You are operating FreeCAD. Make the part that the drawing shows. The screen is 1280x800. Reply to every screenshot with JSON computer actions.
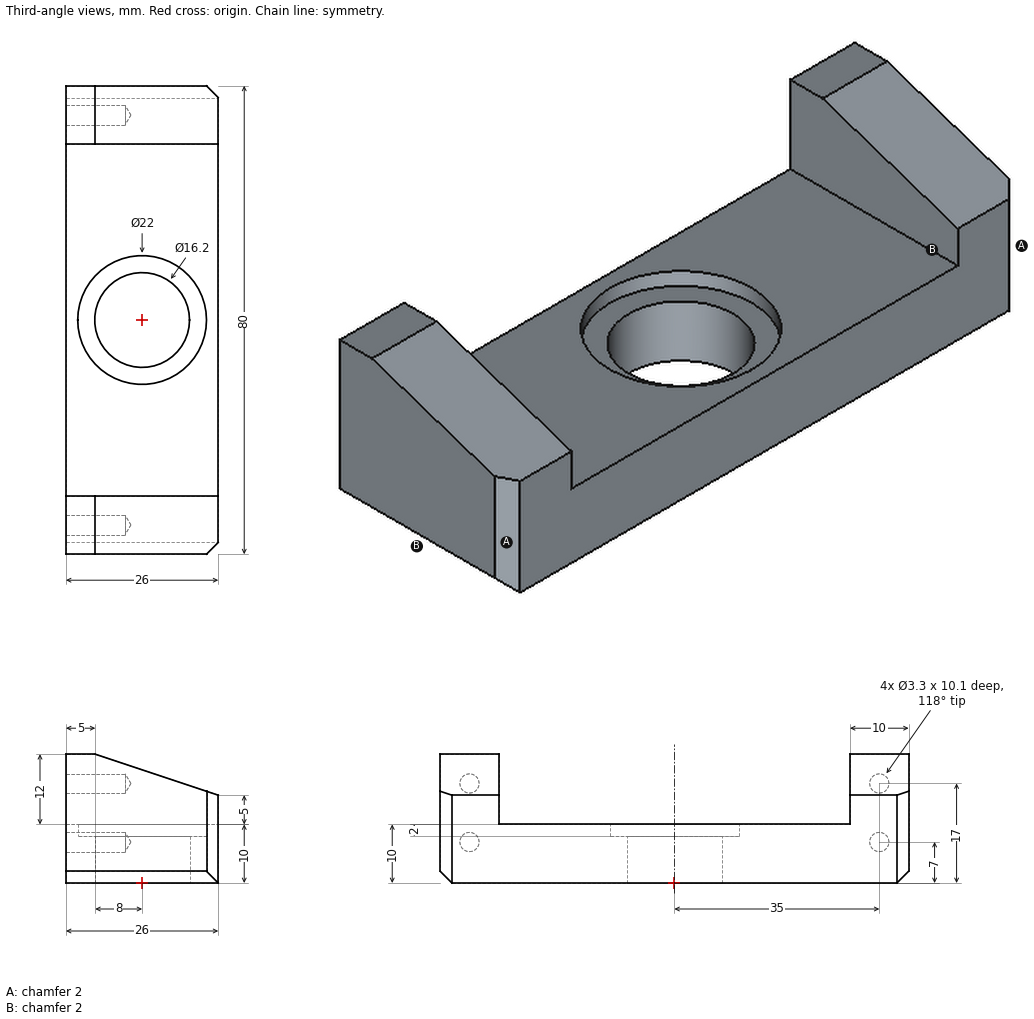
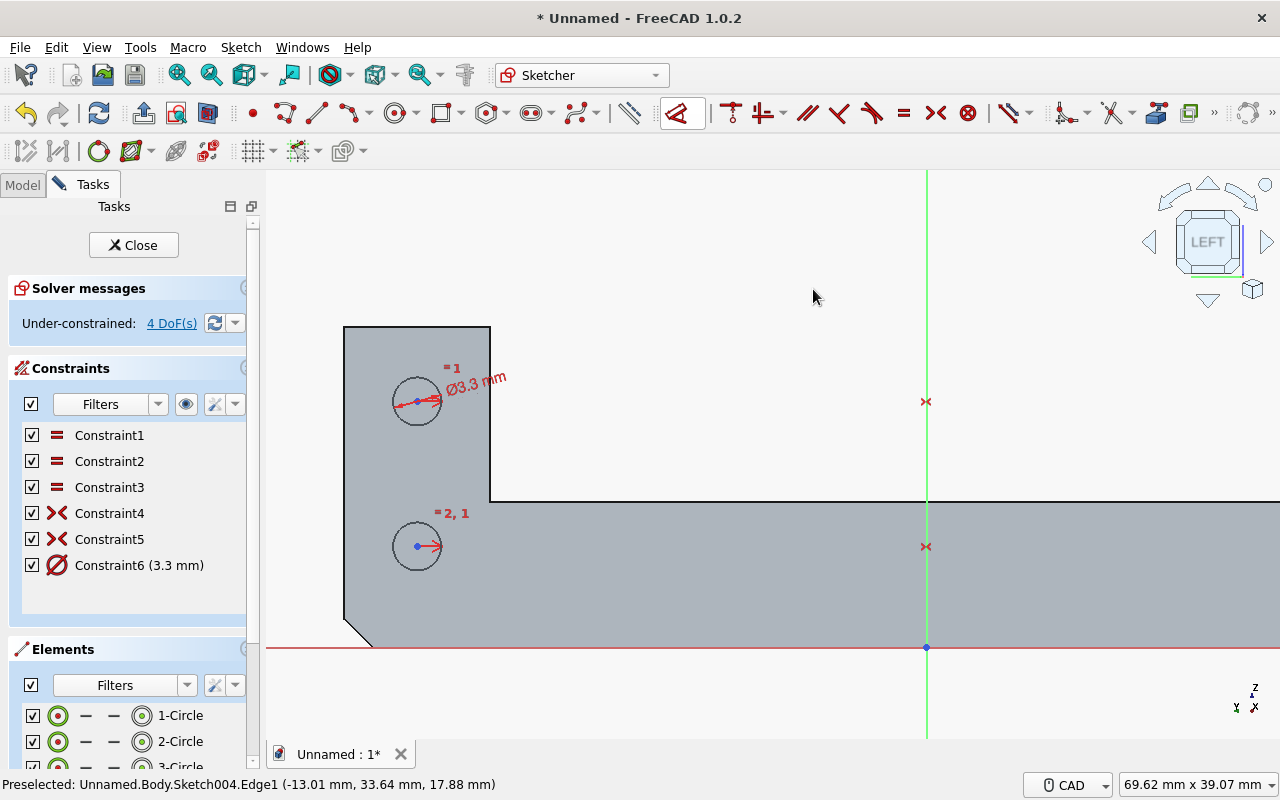
{"action": "left_click", "coordinate": [417, 546]}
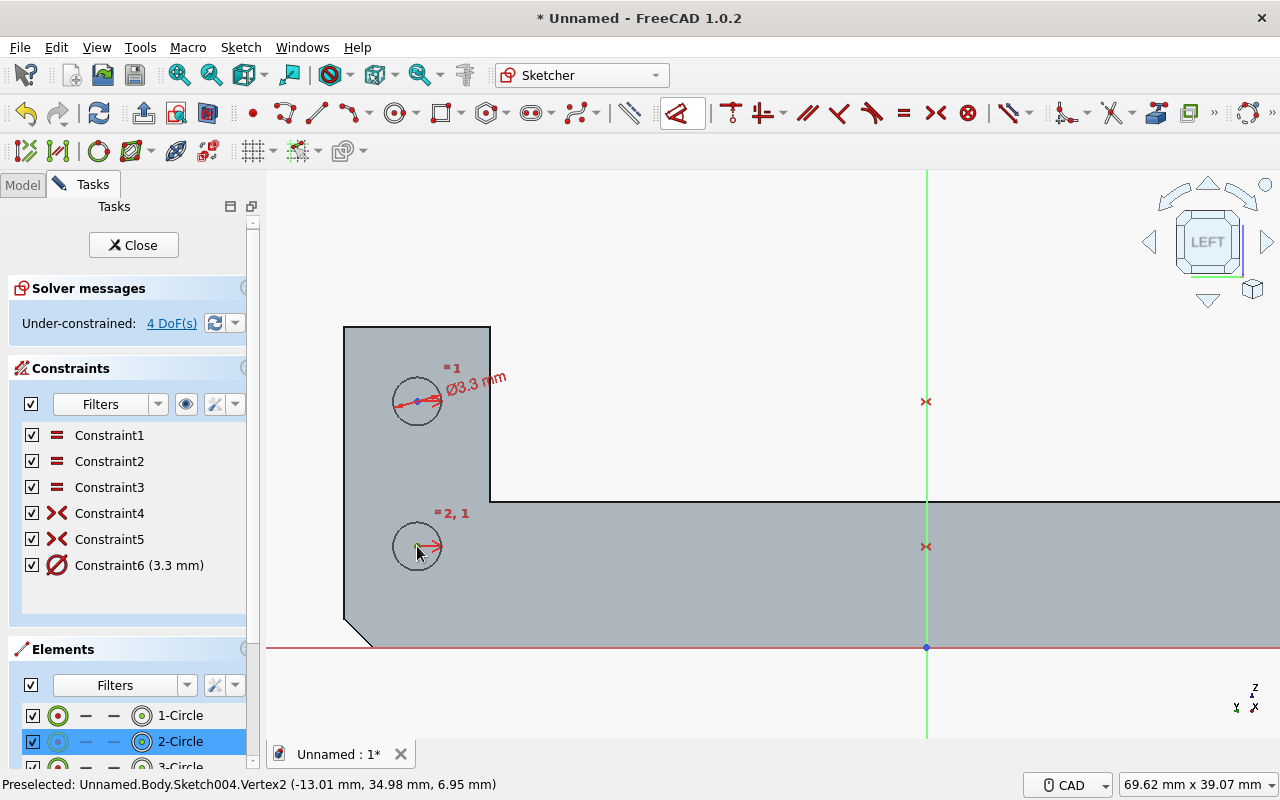
{"action": "key", "text": "i"}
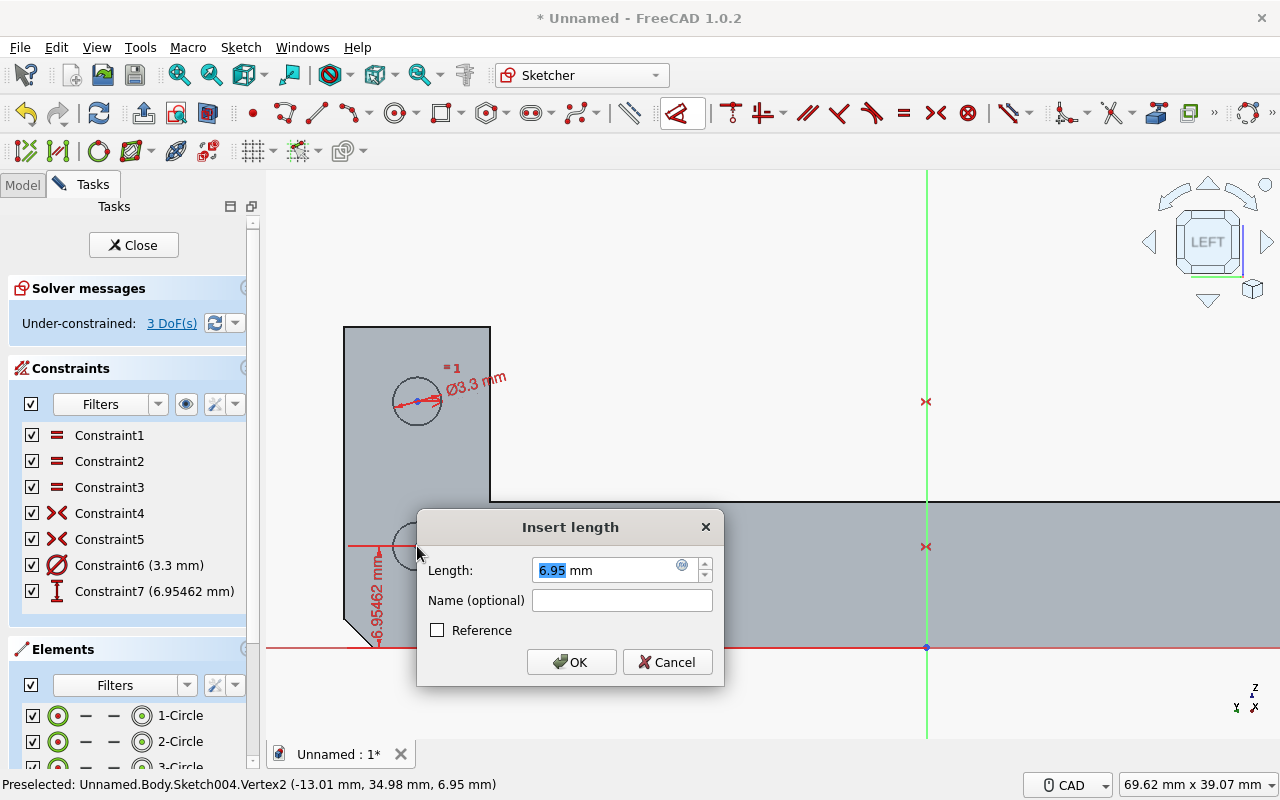
{"action": "type", "text": "7"}
{"action": "key", "text": "Return"}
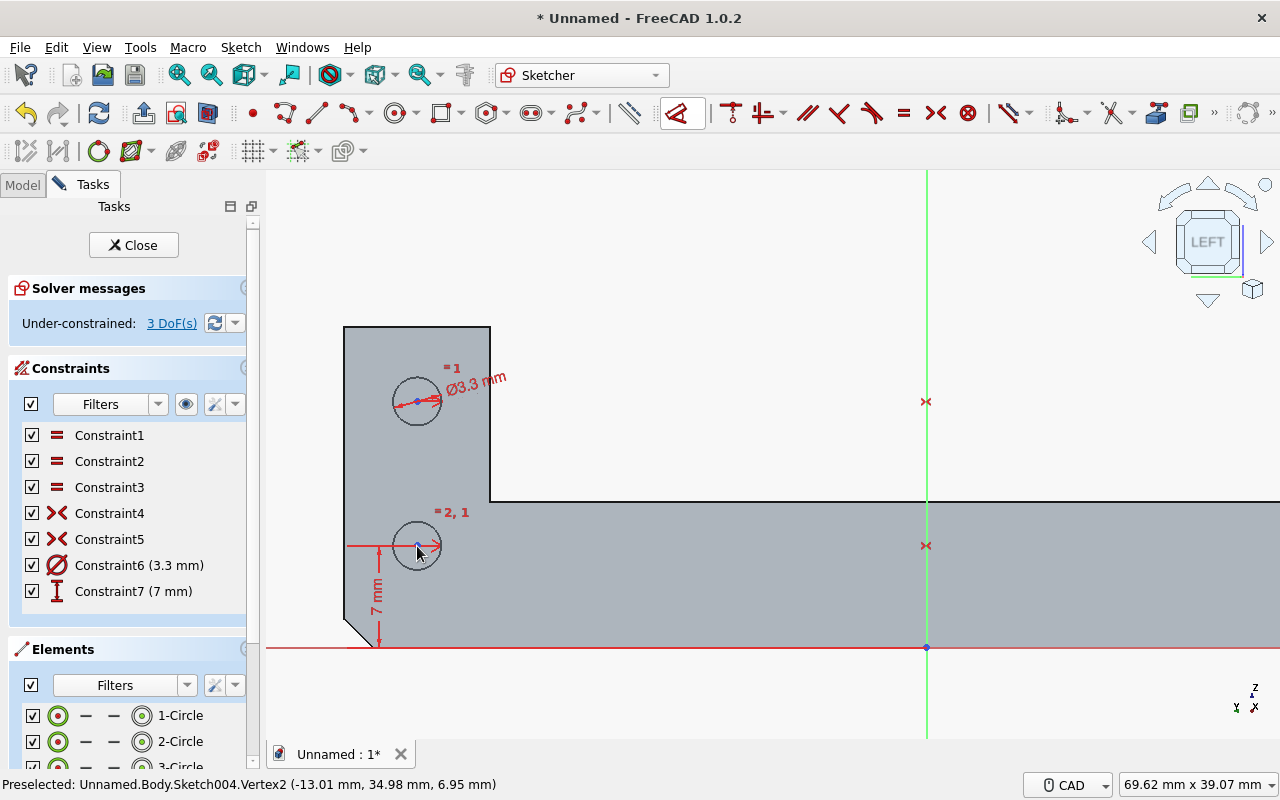
{"action": "left_click", "coordinate": [417, 401]}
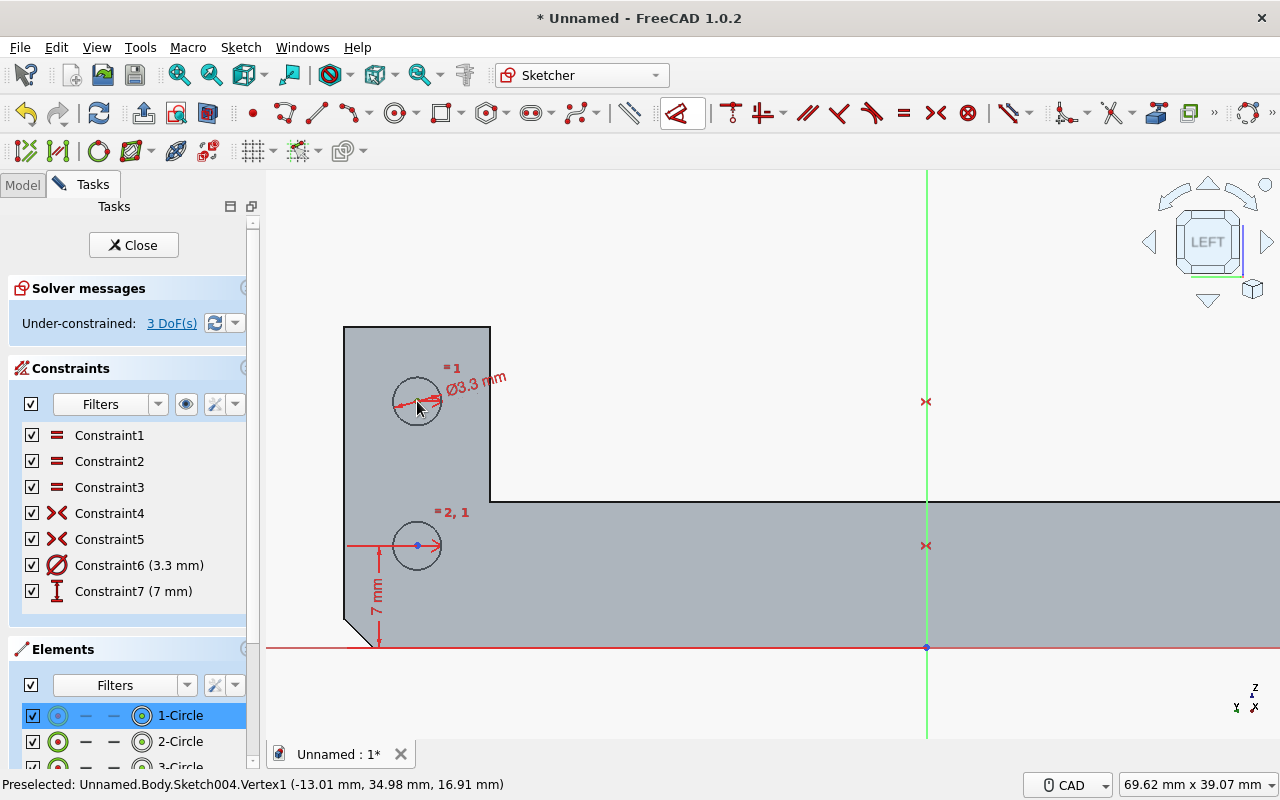
{"action": "left_click", "coordinate": [700, 114]}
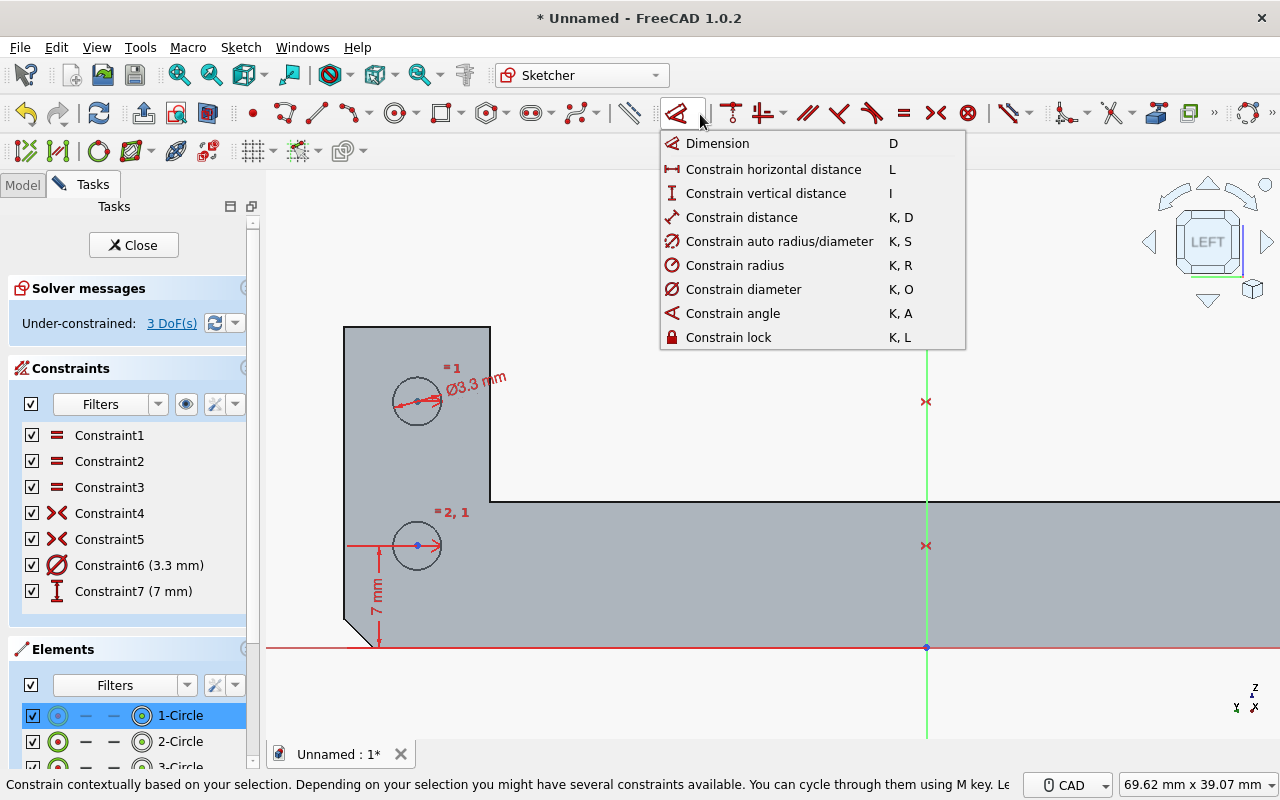
{"action": "left_click", "coordinate": [813, 169]}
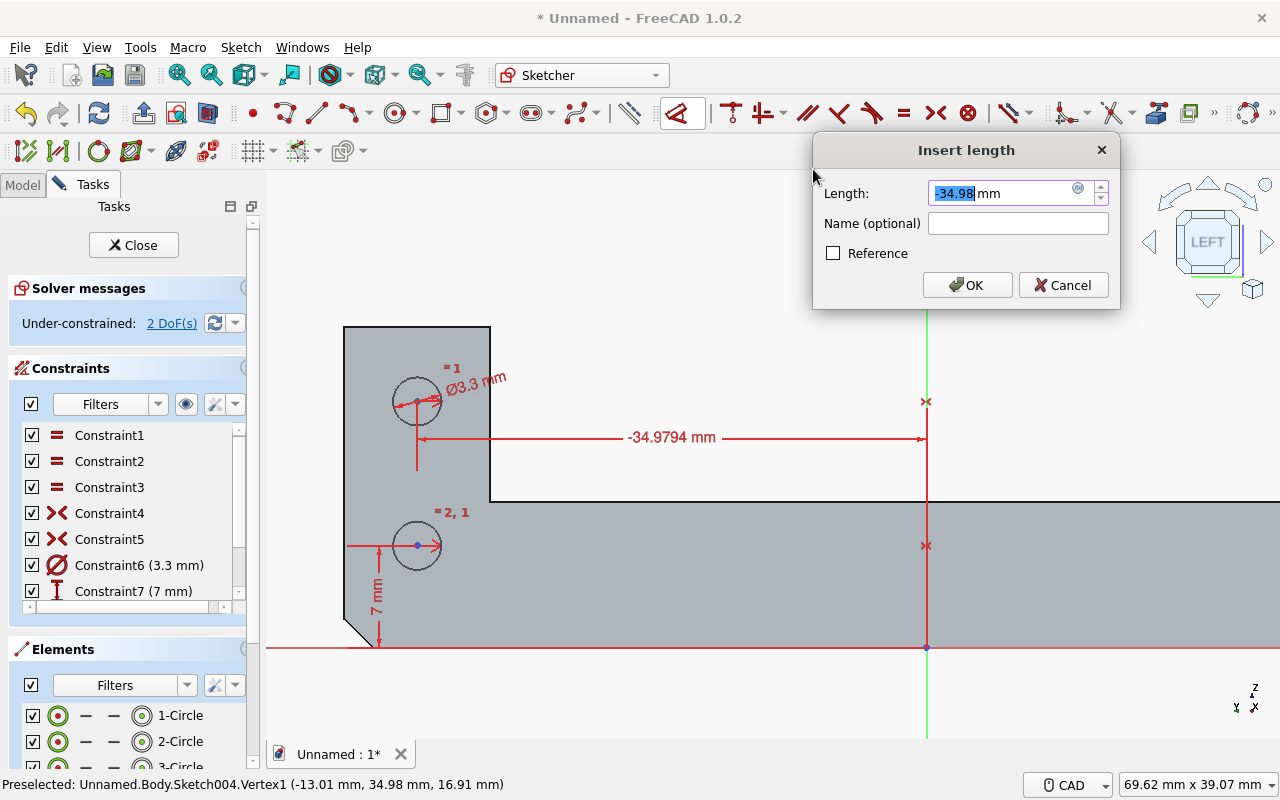
{"action": "type", "text": "-35"}
{"action": "key", "text": "Return"}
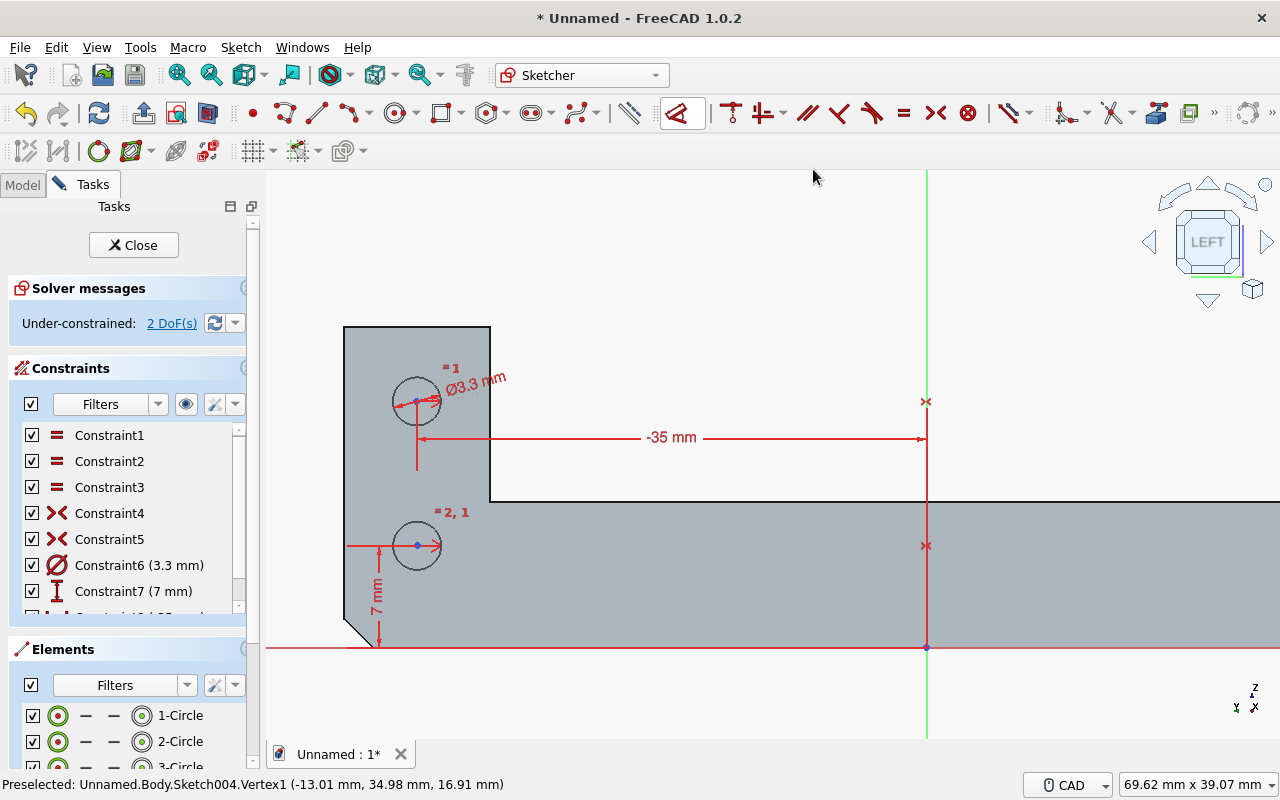
{"action": "left_click", "coordinate": [417, 401]}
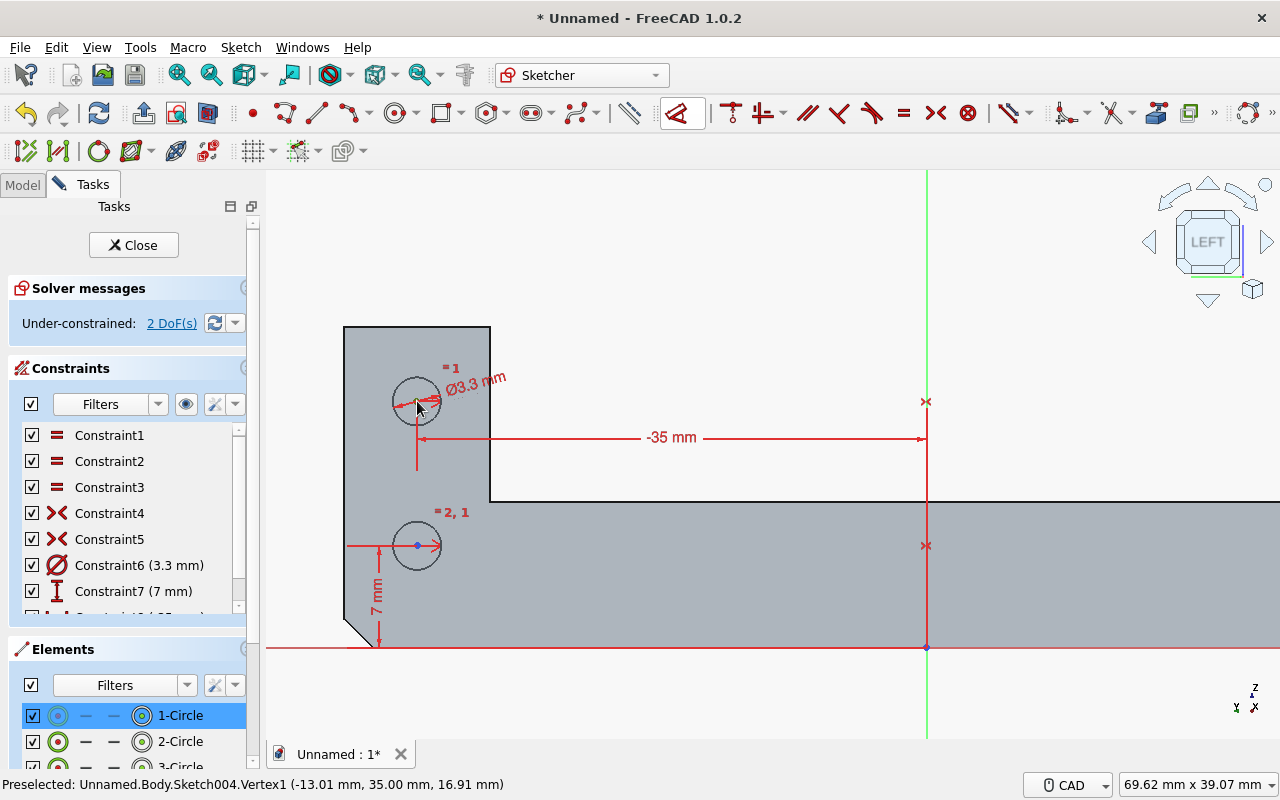
{"action": "key", "text": "i"}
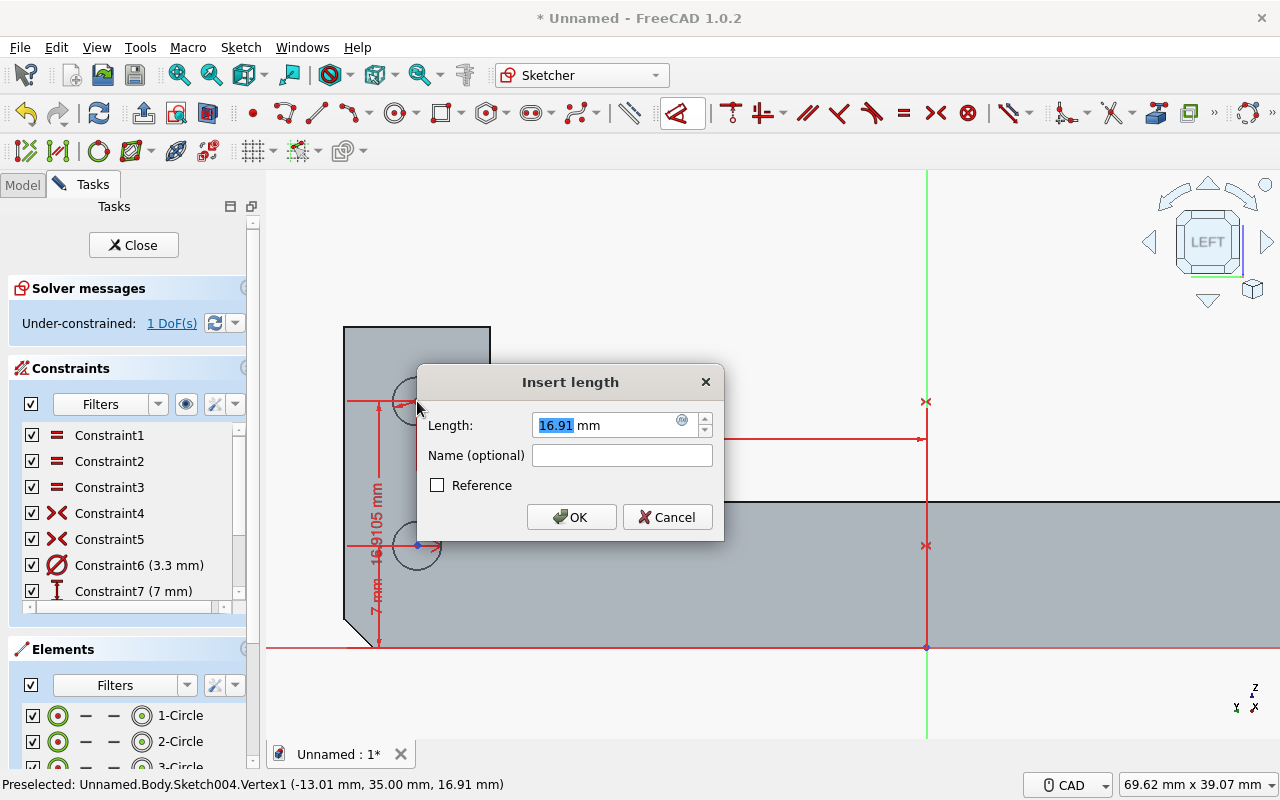
{"action": "type", "text": "17"}
{"action": "key", "text": "Return"}